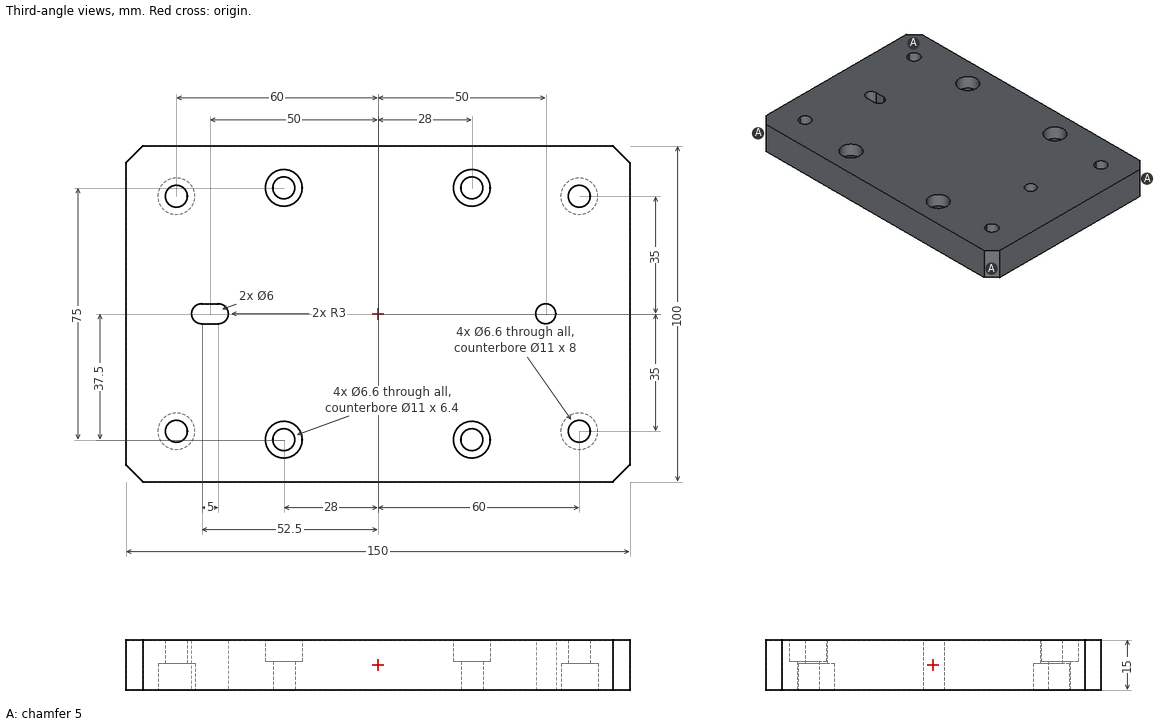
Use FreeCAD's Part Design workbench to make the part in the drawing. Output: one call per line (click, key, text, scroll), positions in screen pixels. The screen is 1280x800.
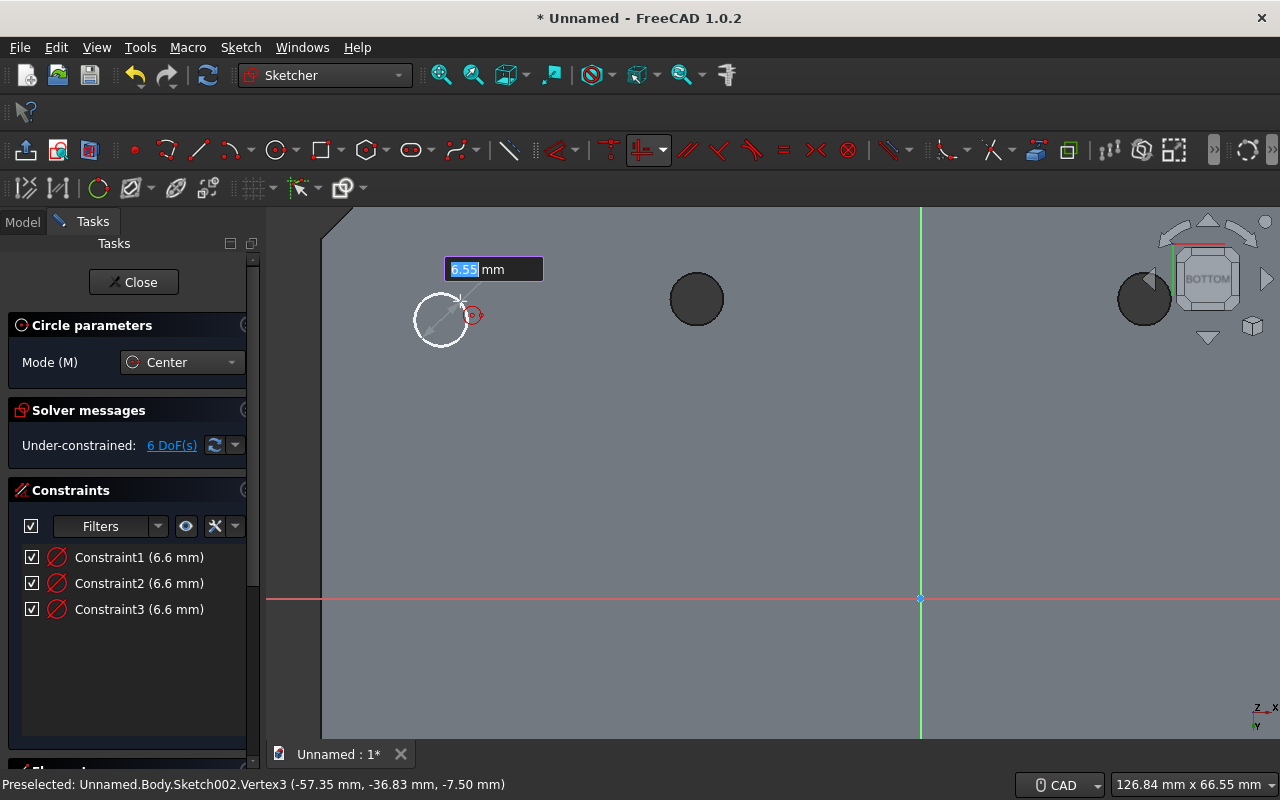
text(6.6)
key(Return)
key(Escape)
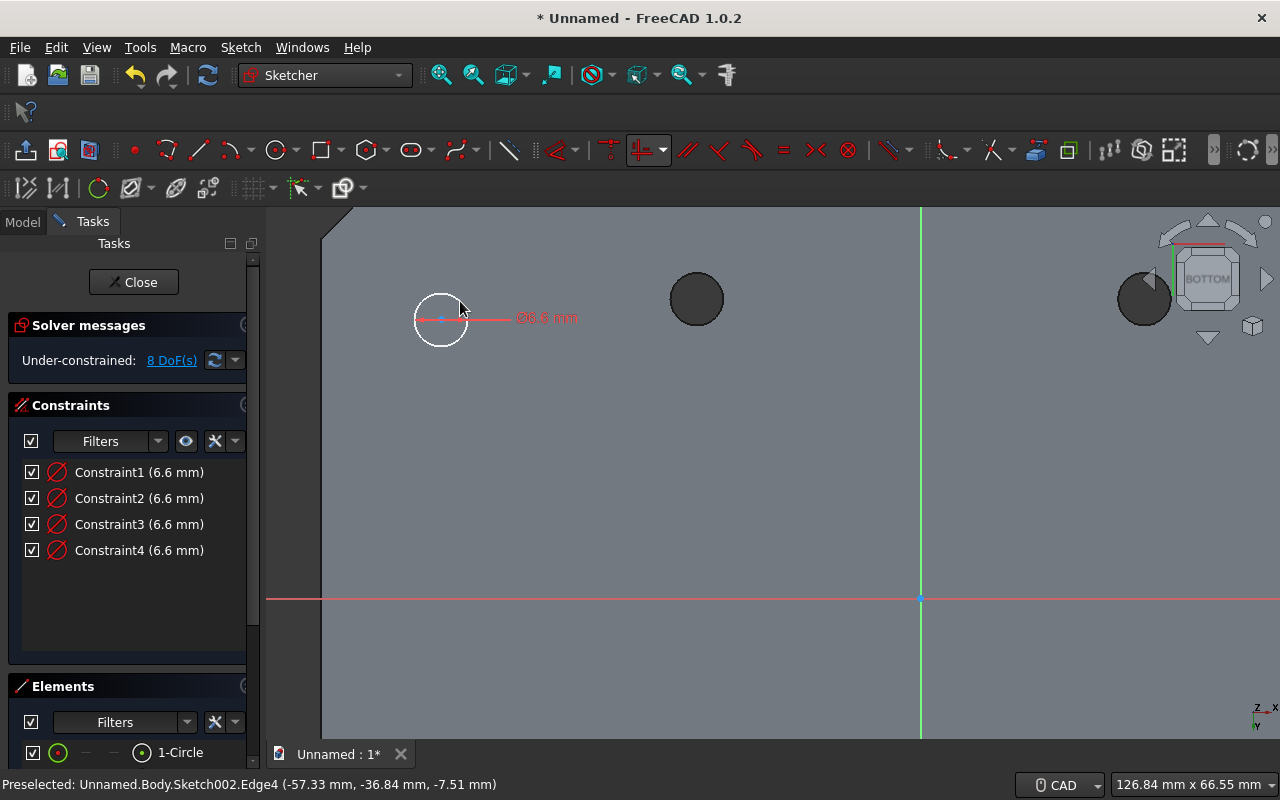
scroll(442, 320, down, 3)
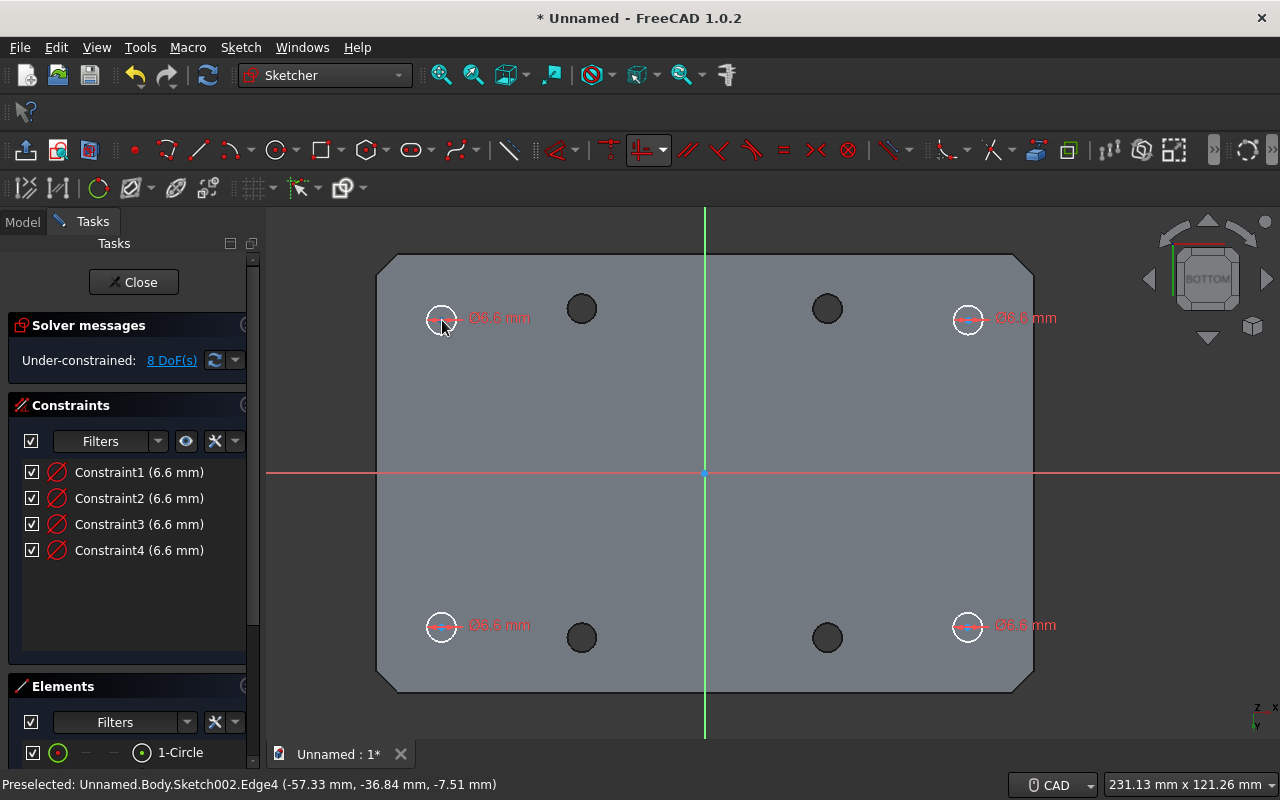
click(968, 320)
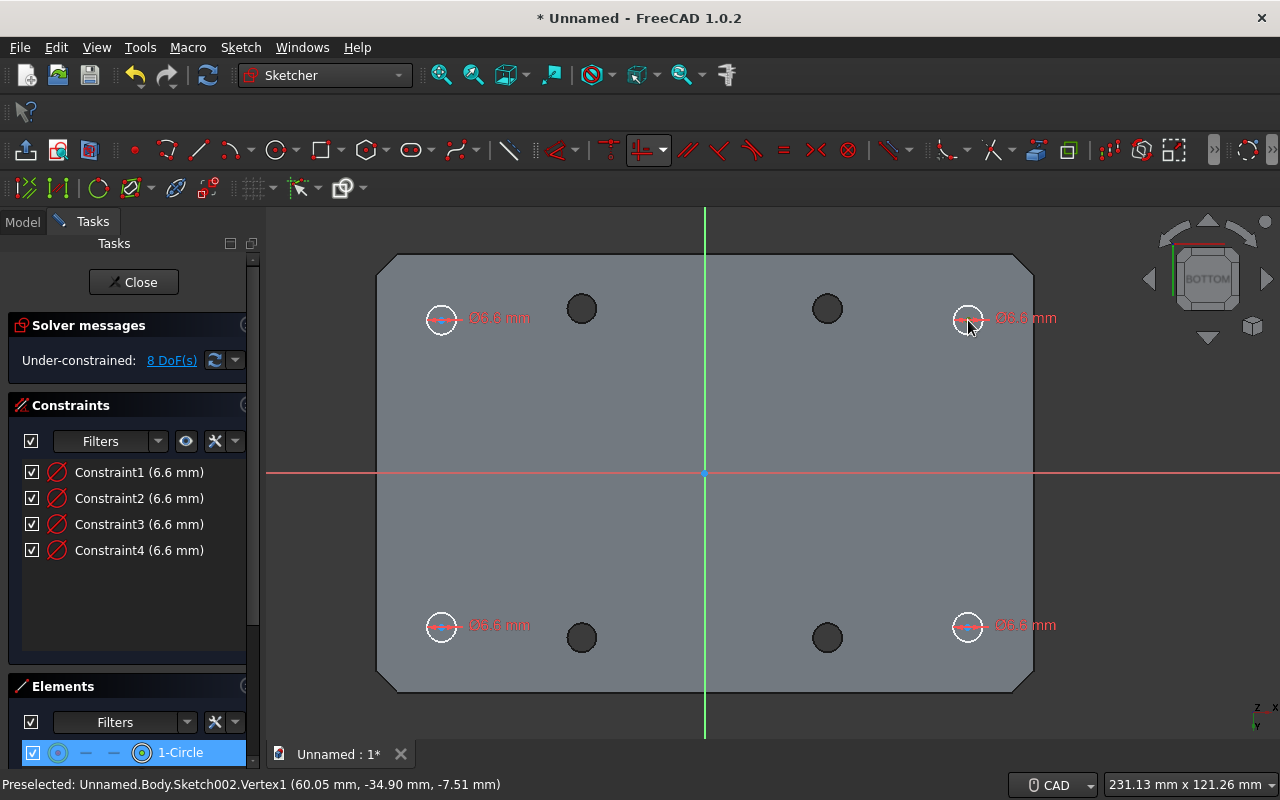
click(968, 627)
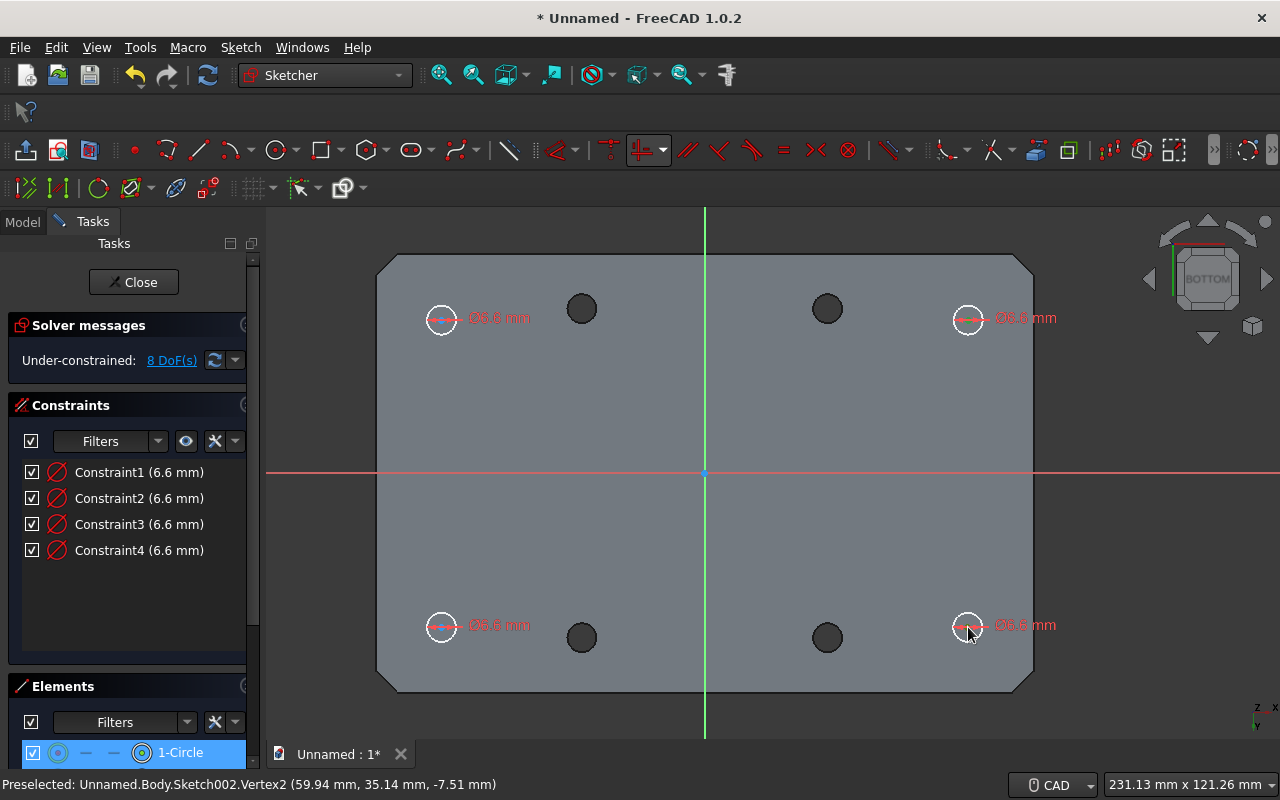
key(v)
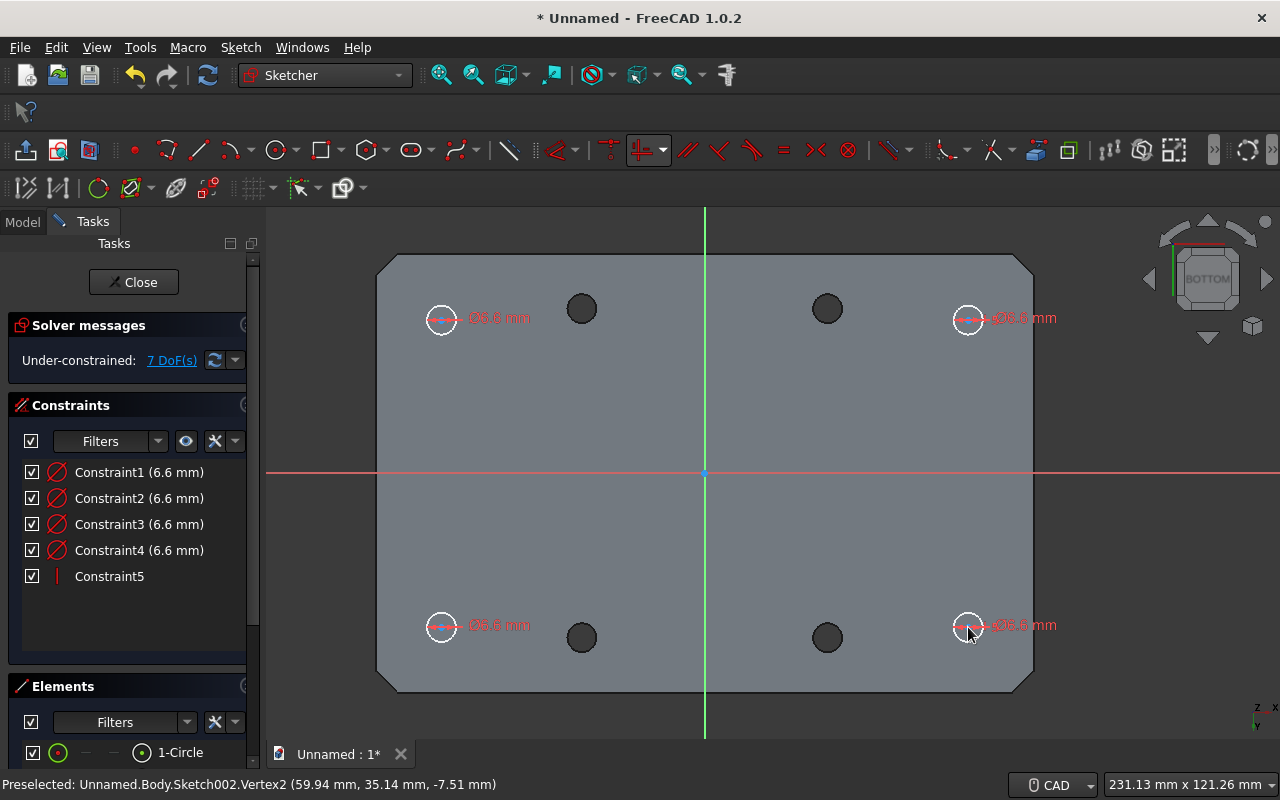
click(968, 627)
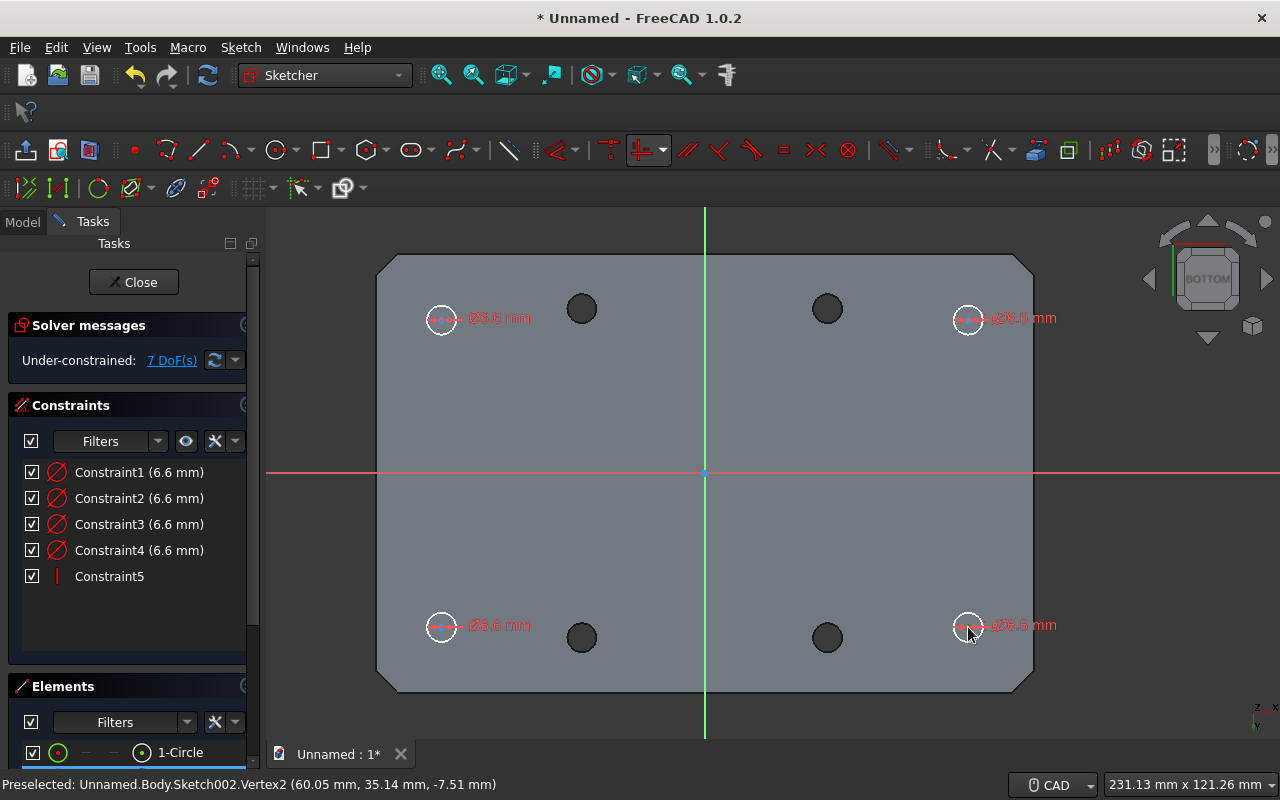
click(442, 627)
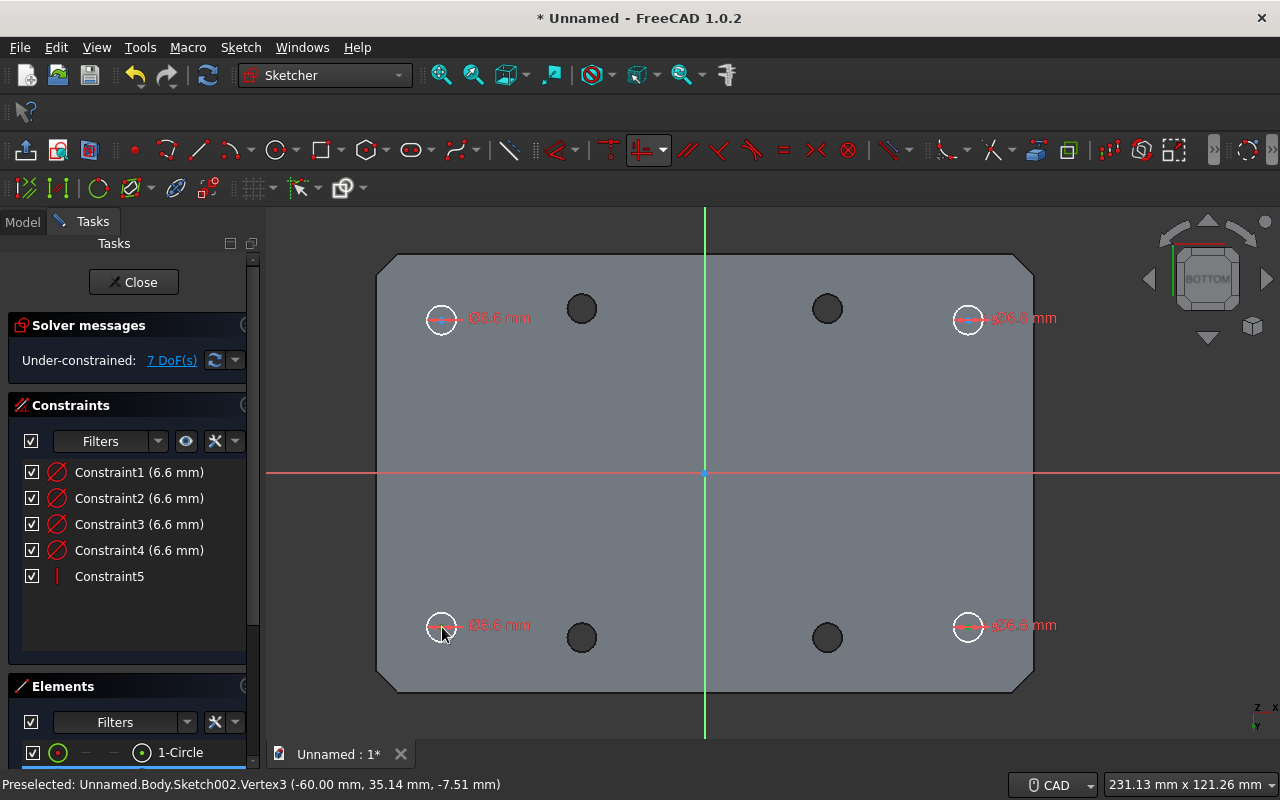
key(h)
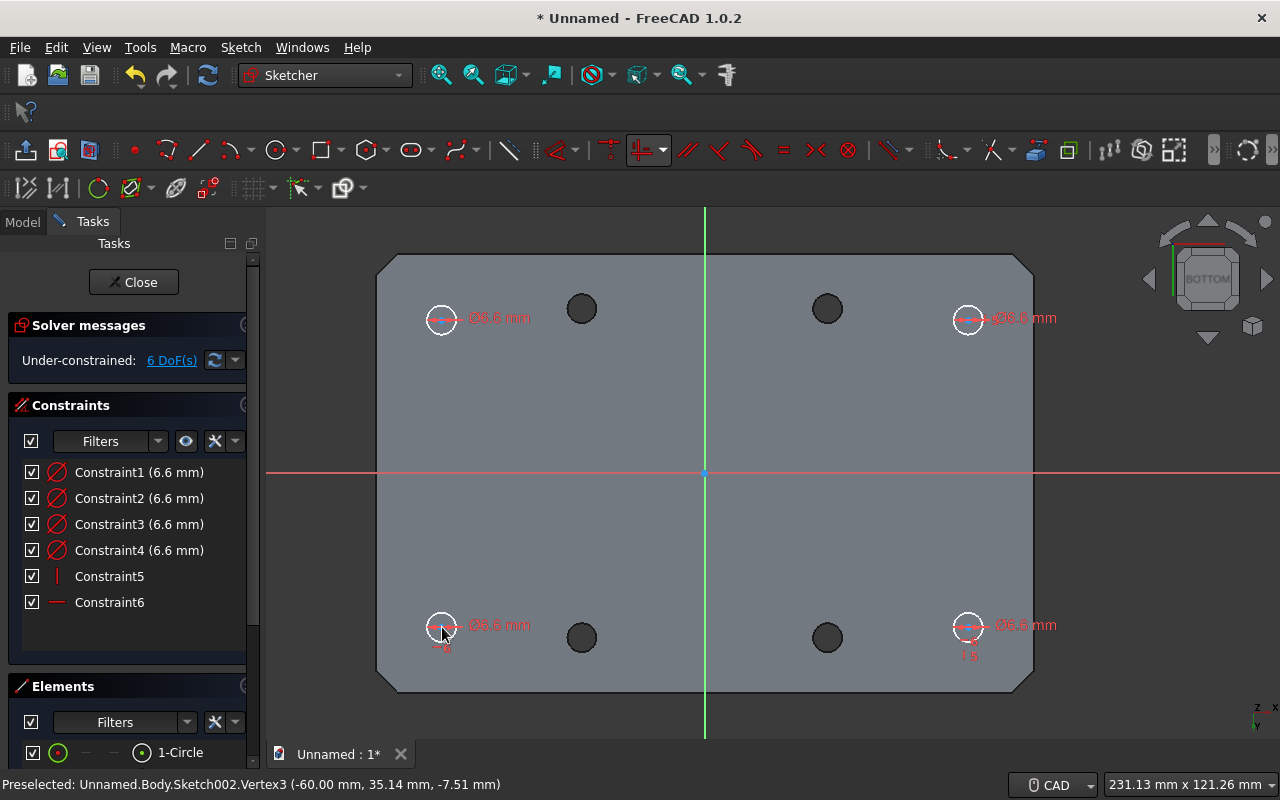
click(442, 627)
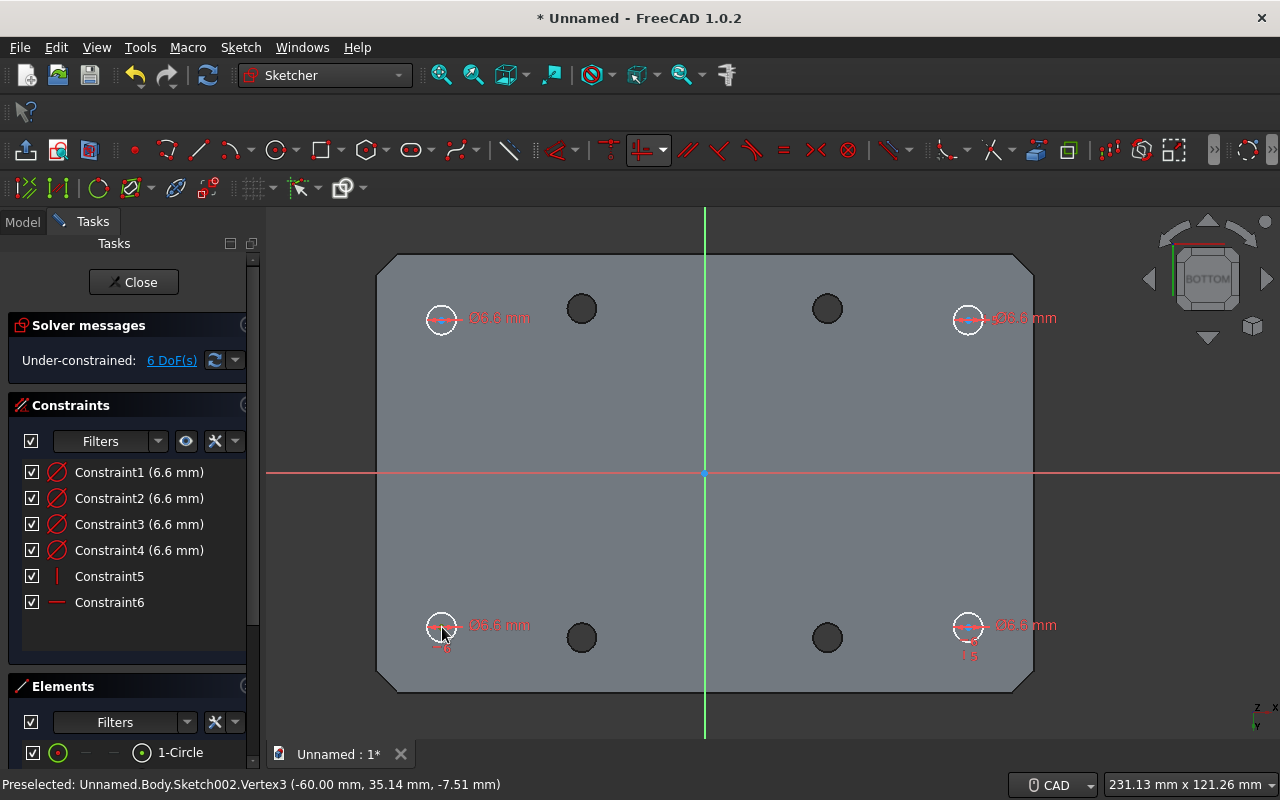
click(442, 320)